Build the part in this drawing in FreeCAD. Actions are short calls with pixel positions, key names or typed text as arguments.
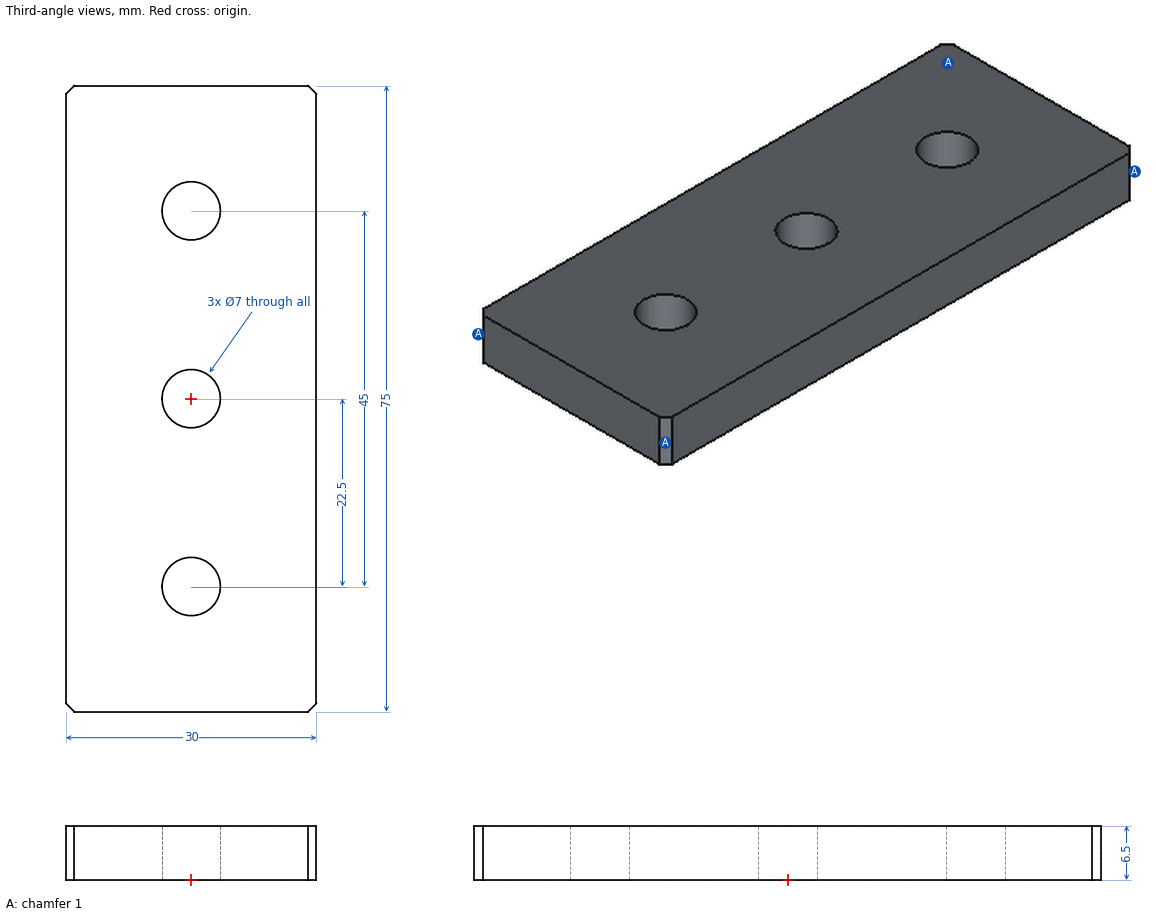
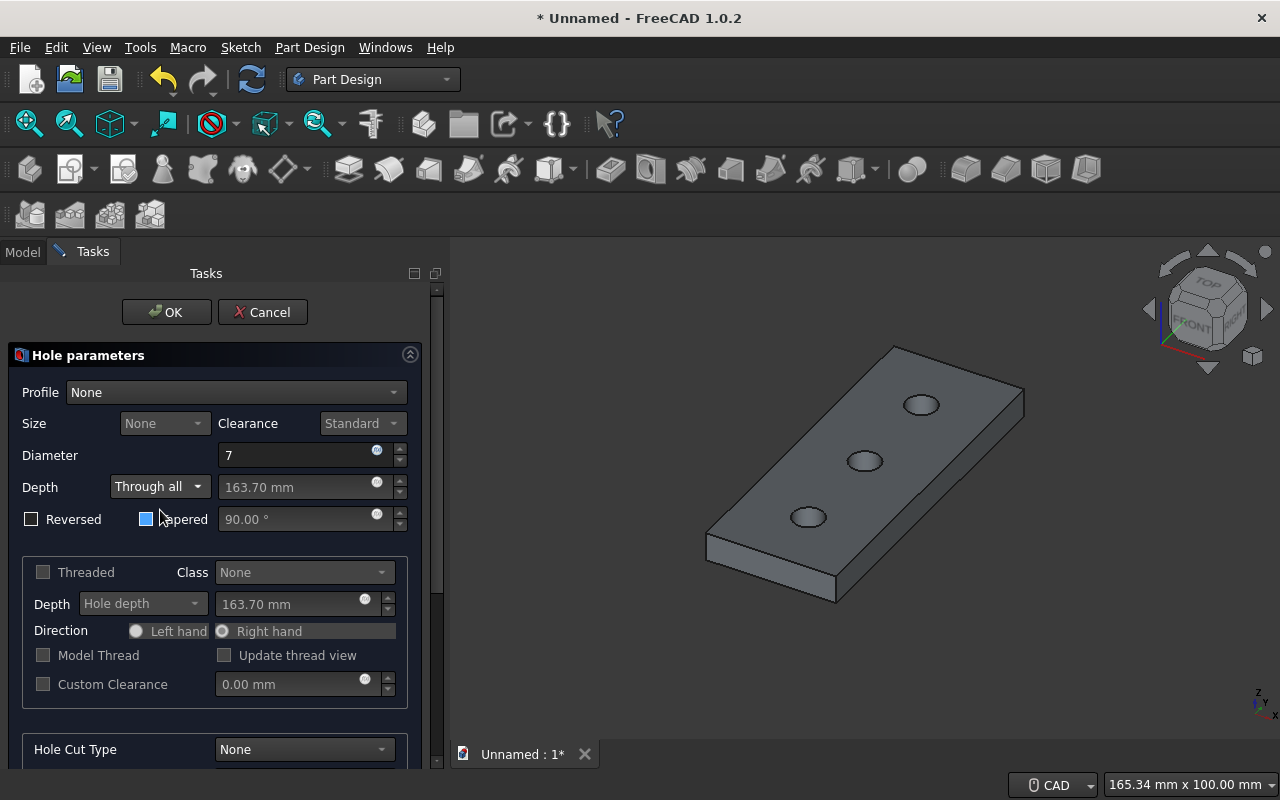
click(167, 312)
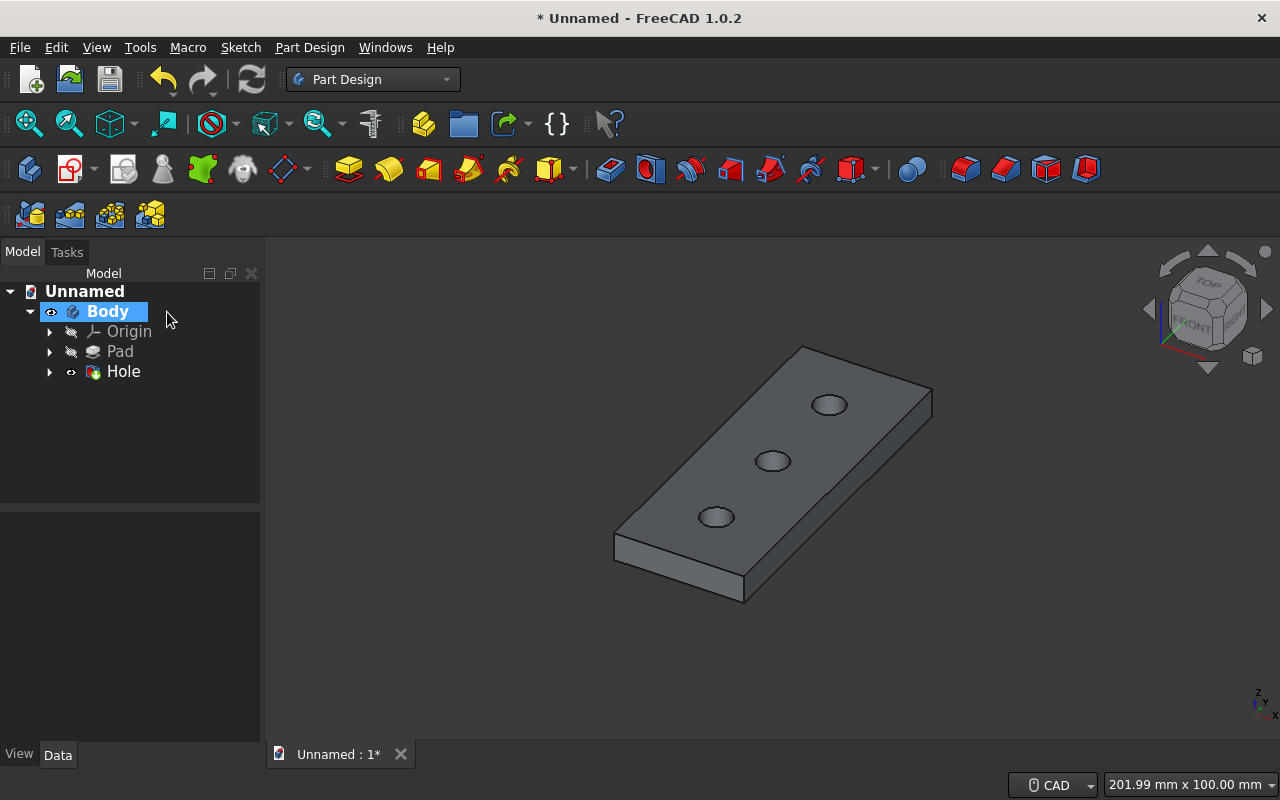
click(744, 589)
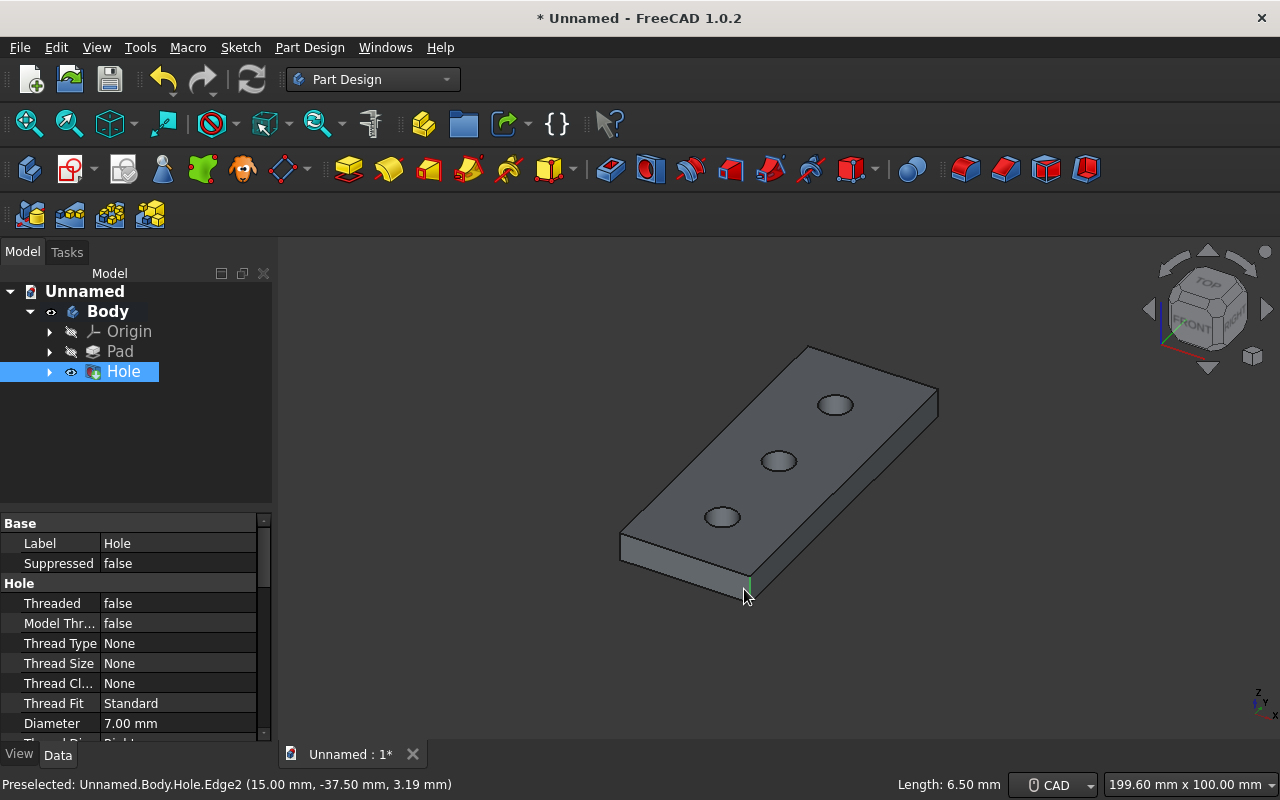
key(0)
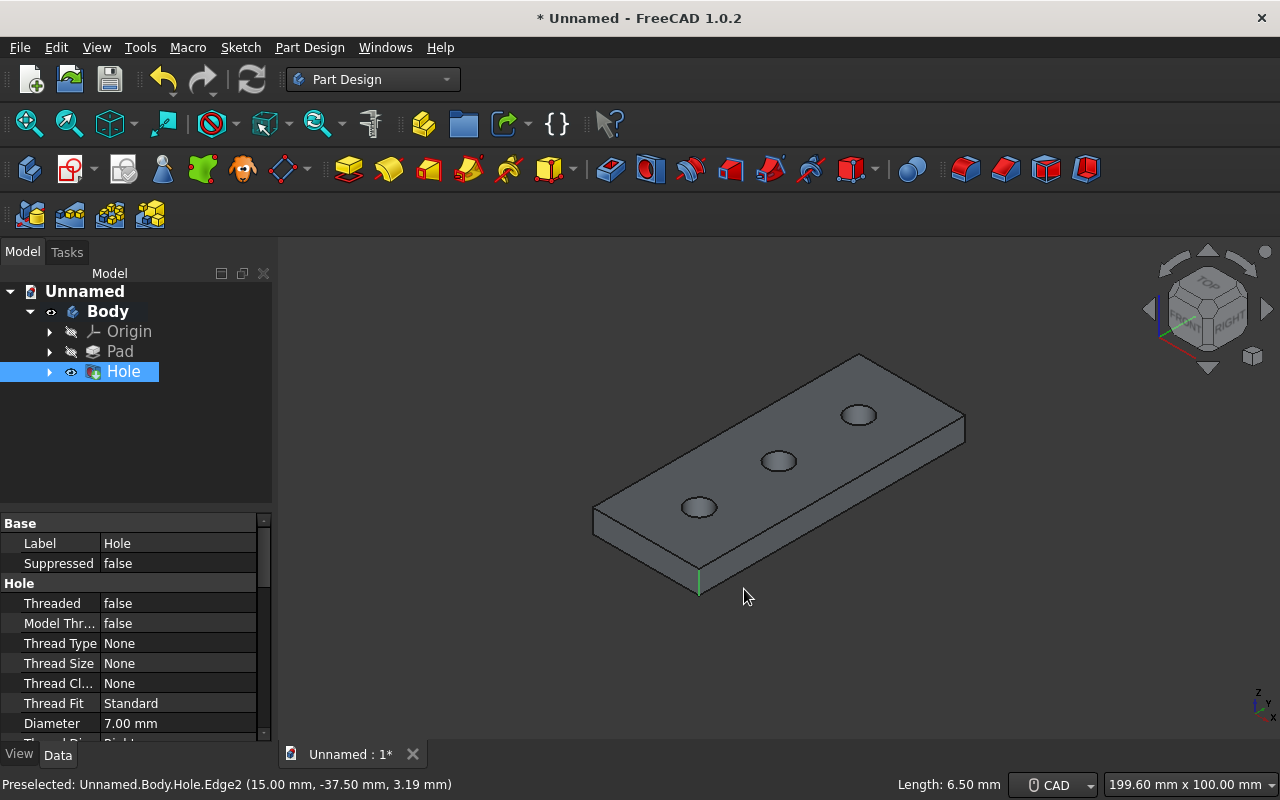
key(2)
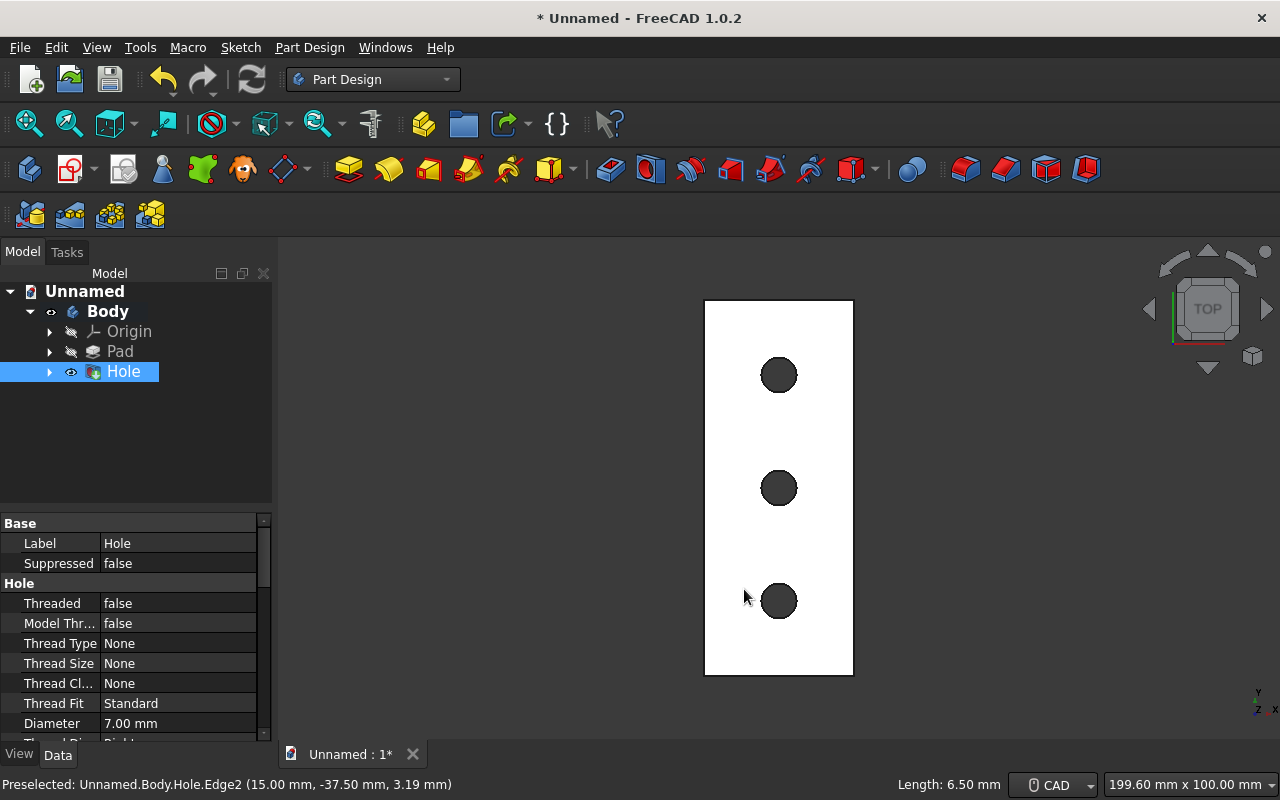
key(1)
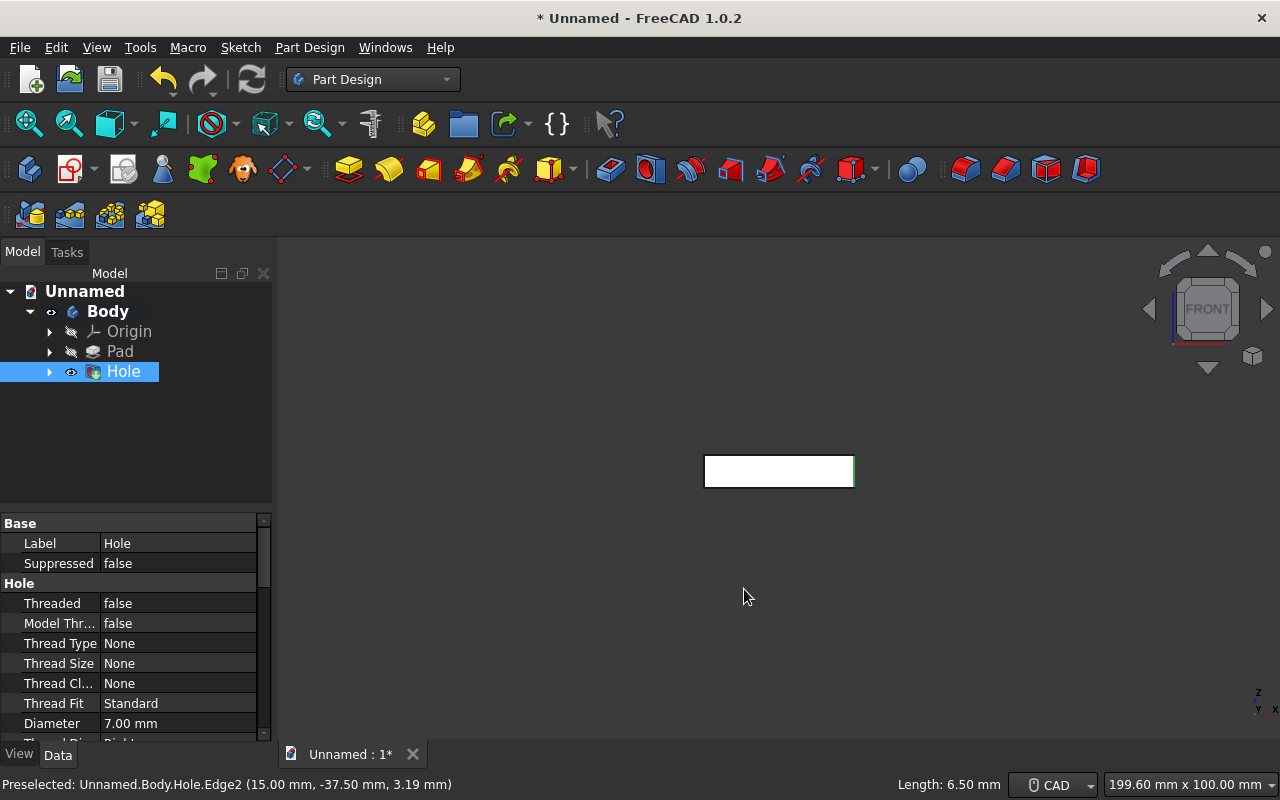
key(v)
key(f)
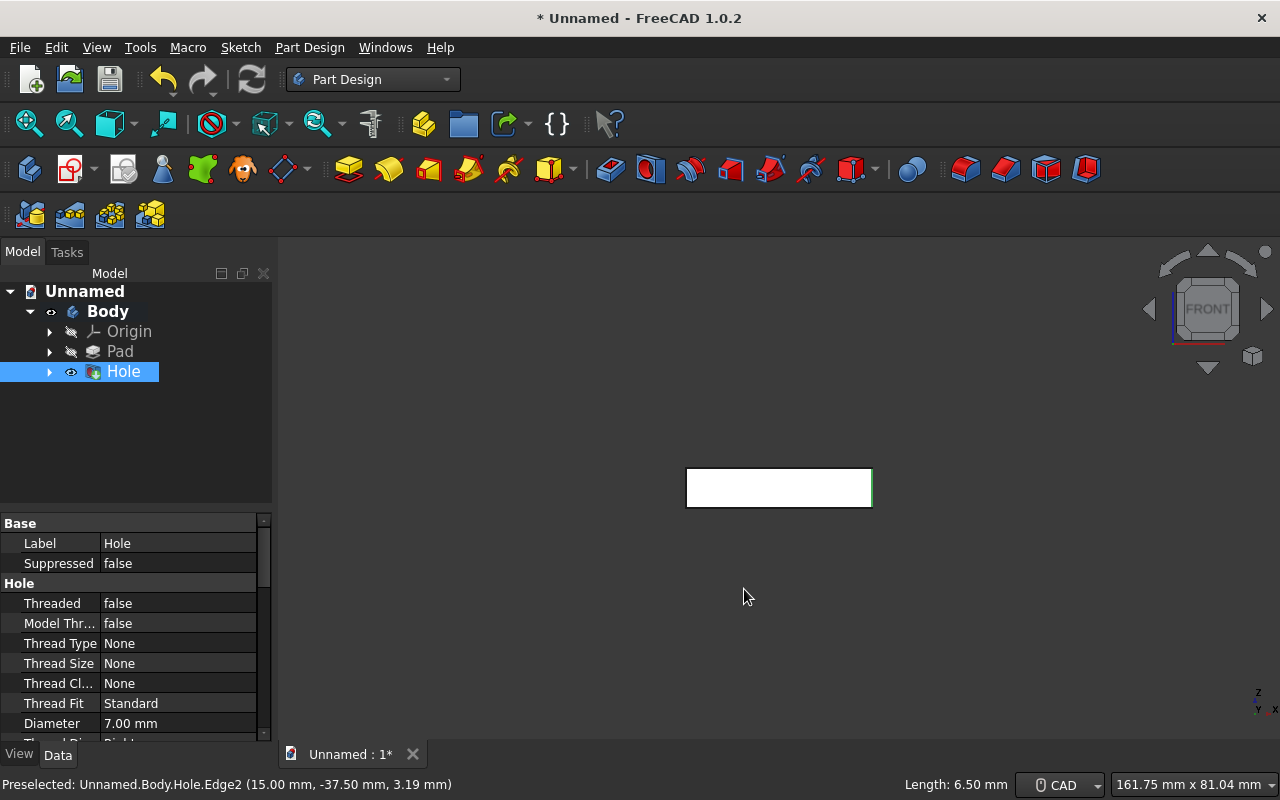
click(686, 487, ctrl)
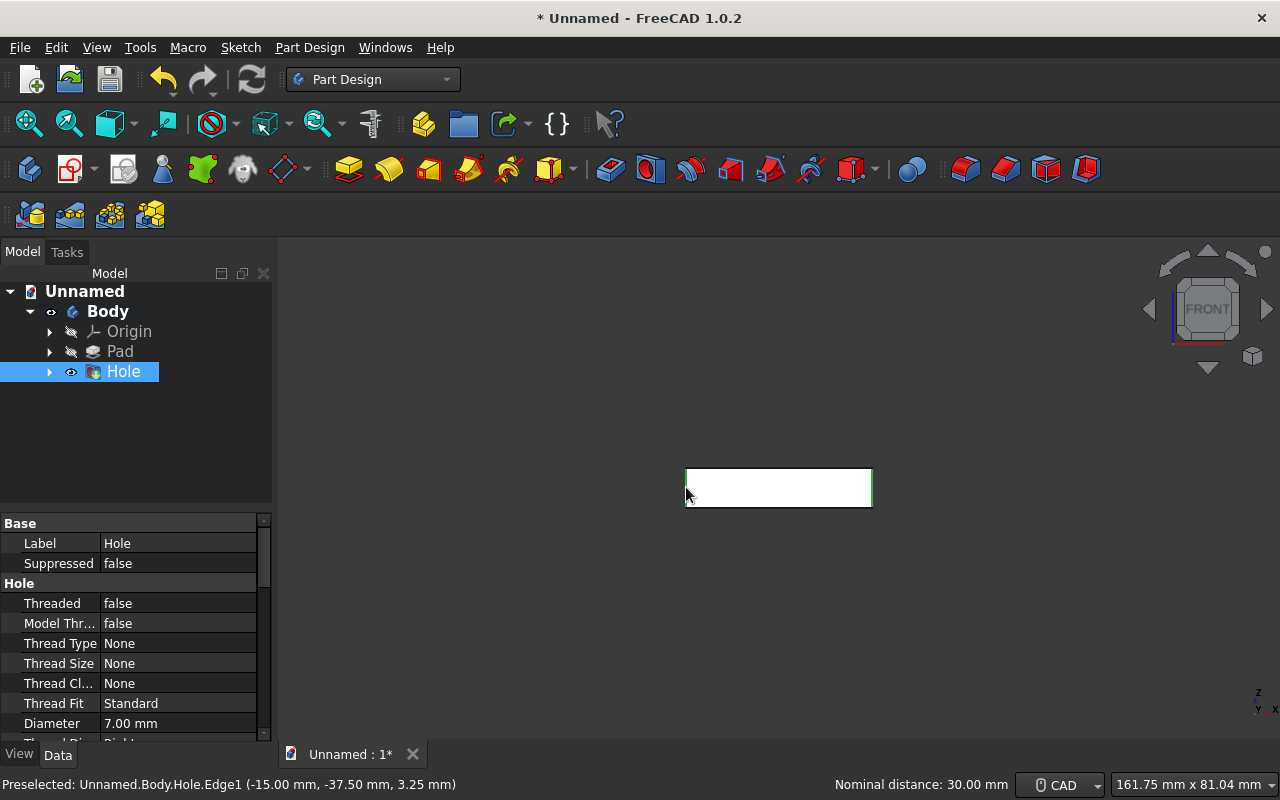
key(3)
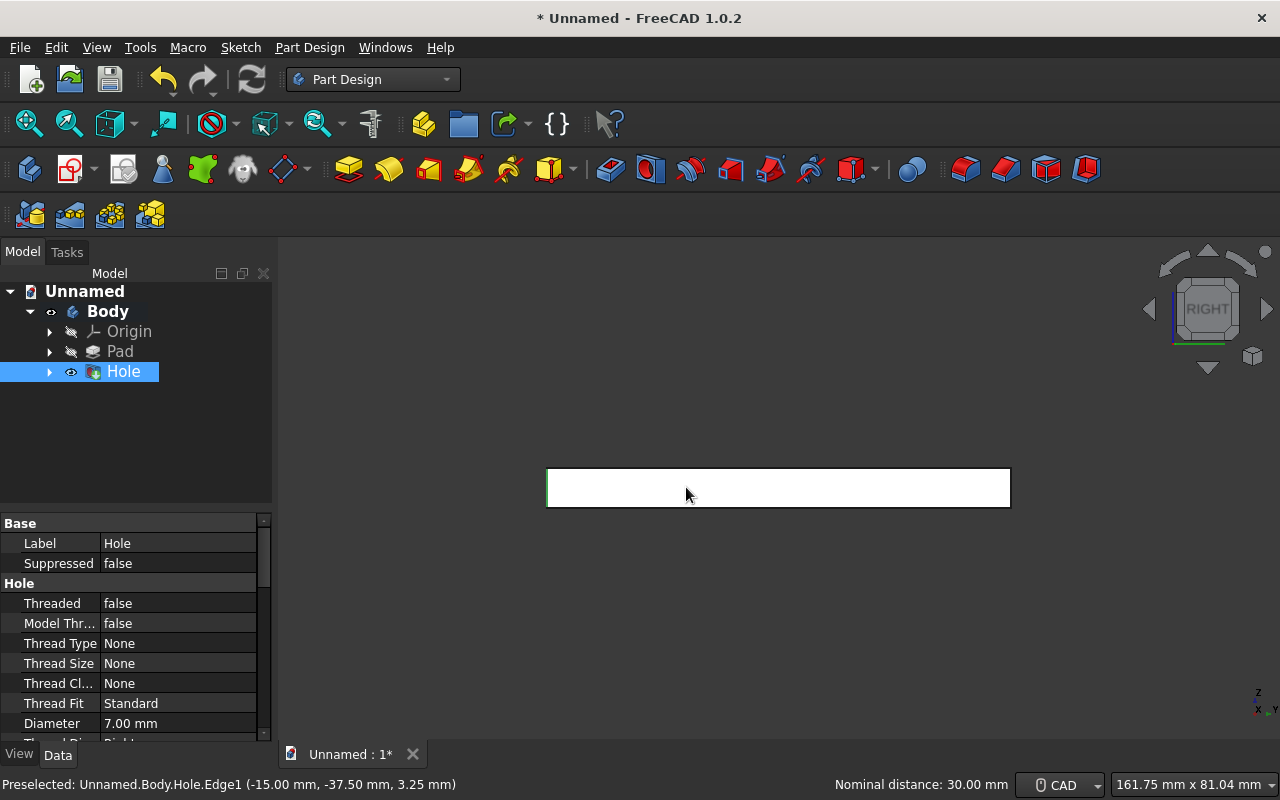
click(1011, 487, ctrl)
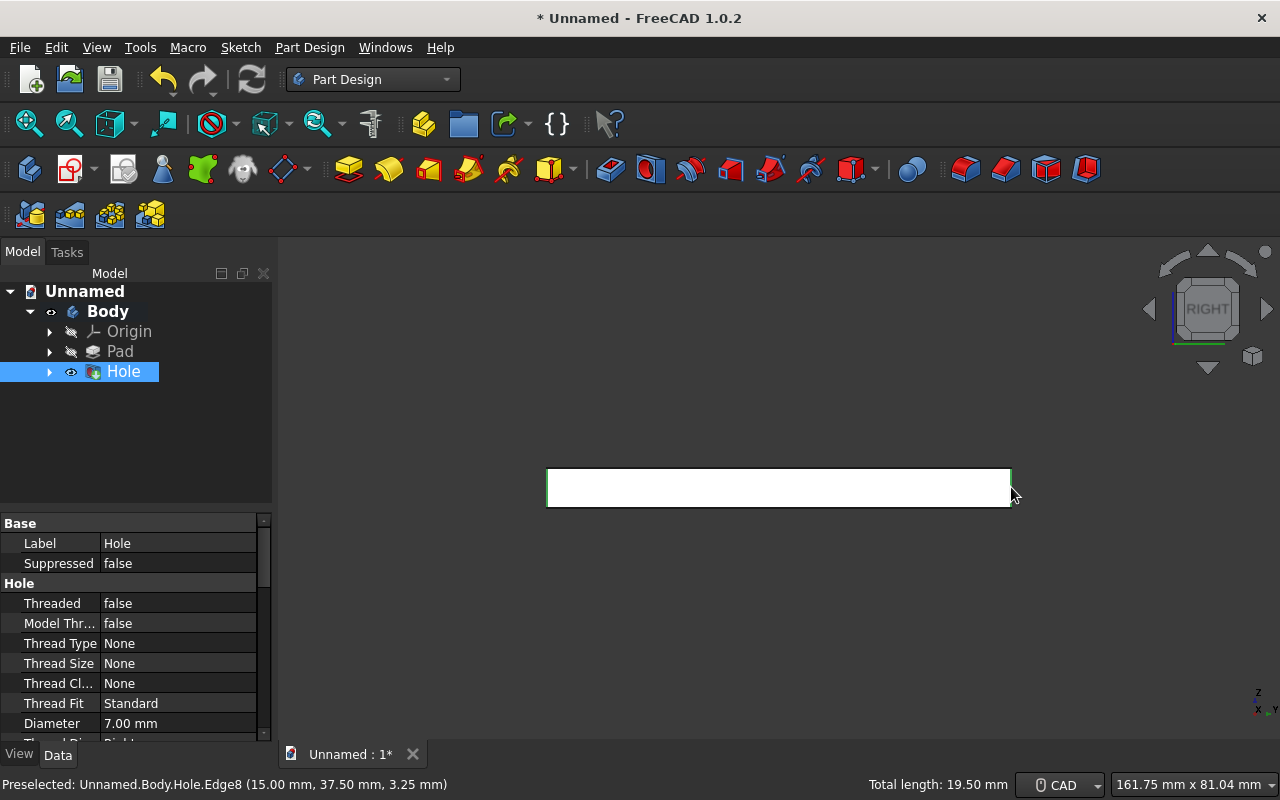
key(5)